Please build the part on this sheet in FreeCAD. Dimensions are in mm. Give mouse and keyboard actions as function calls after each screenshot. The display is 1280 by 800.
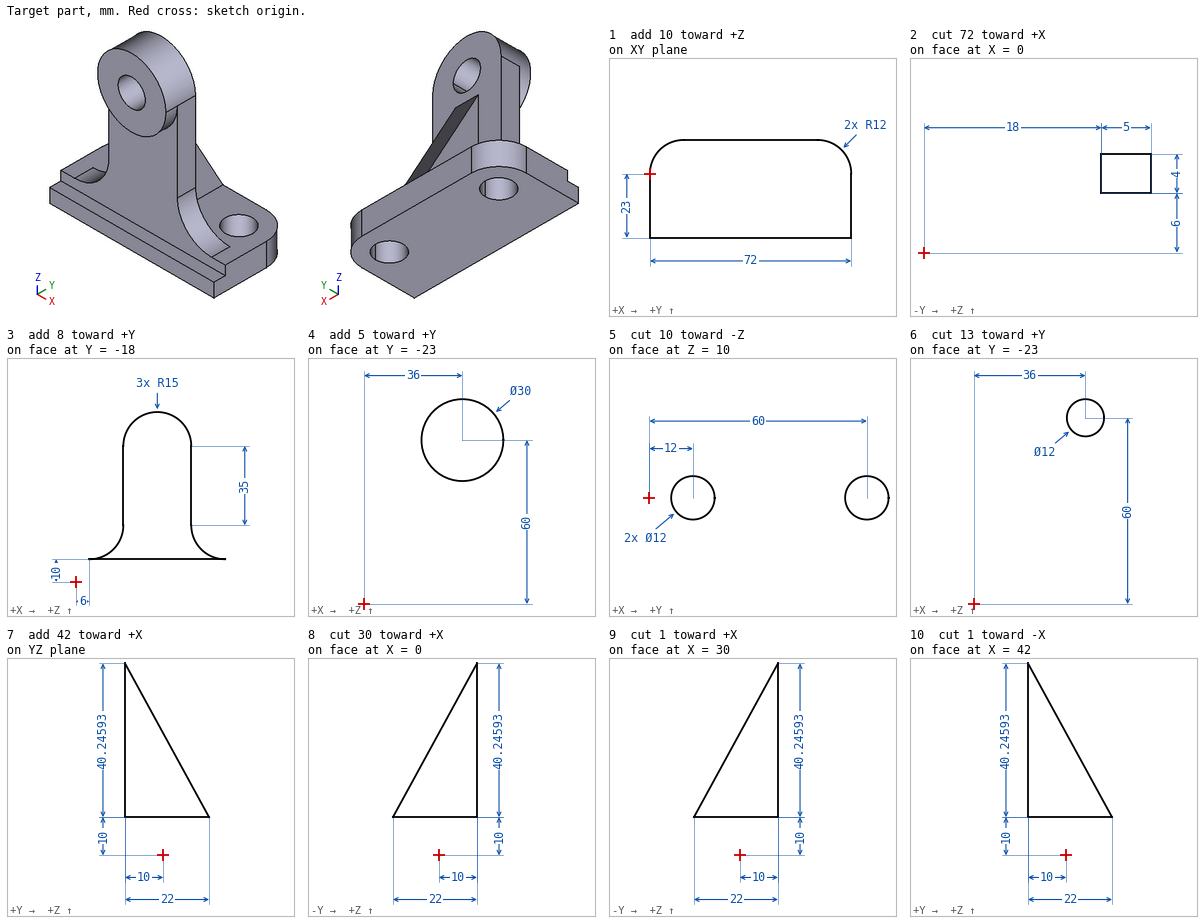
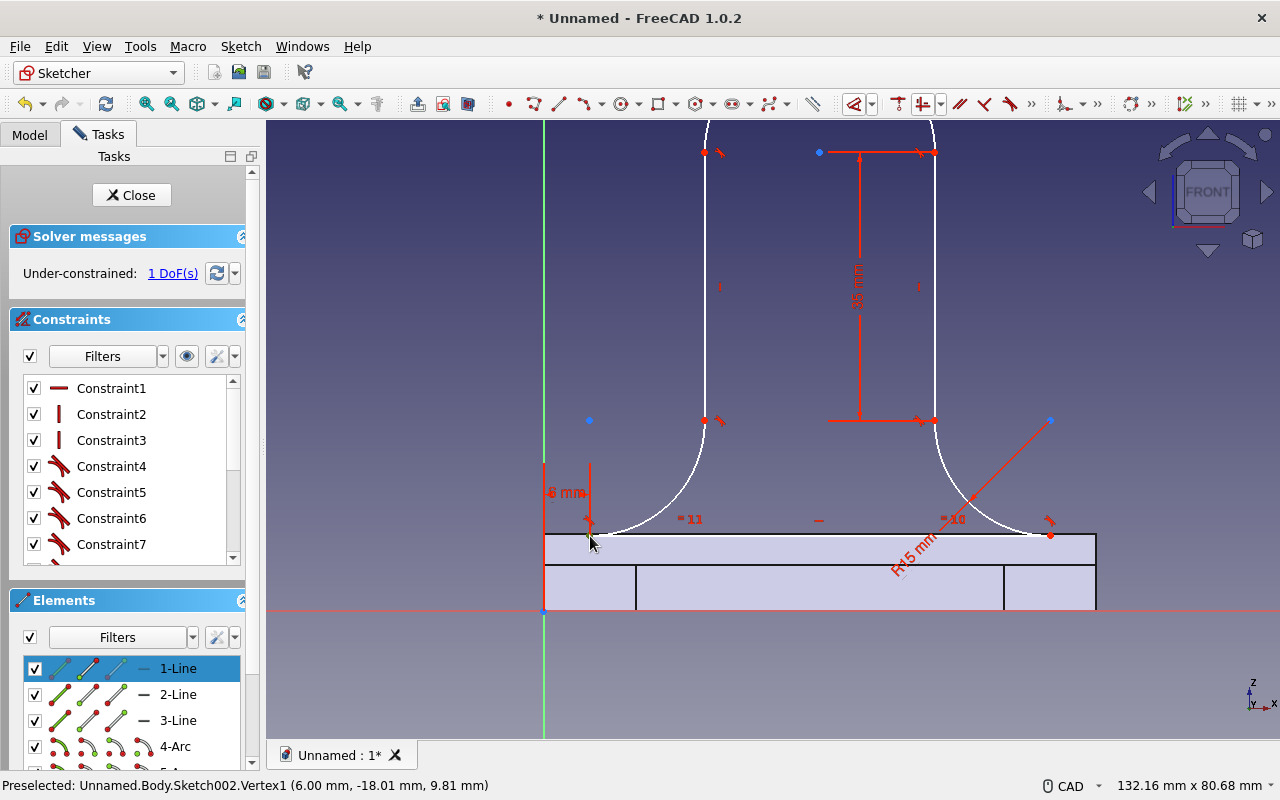
click(872, 104)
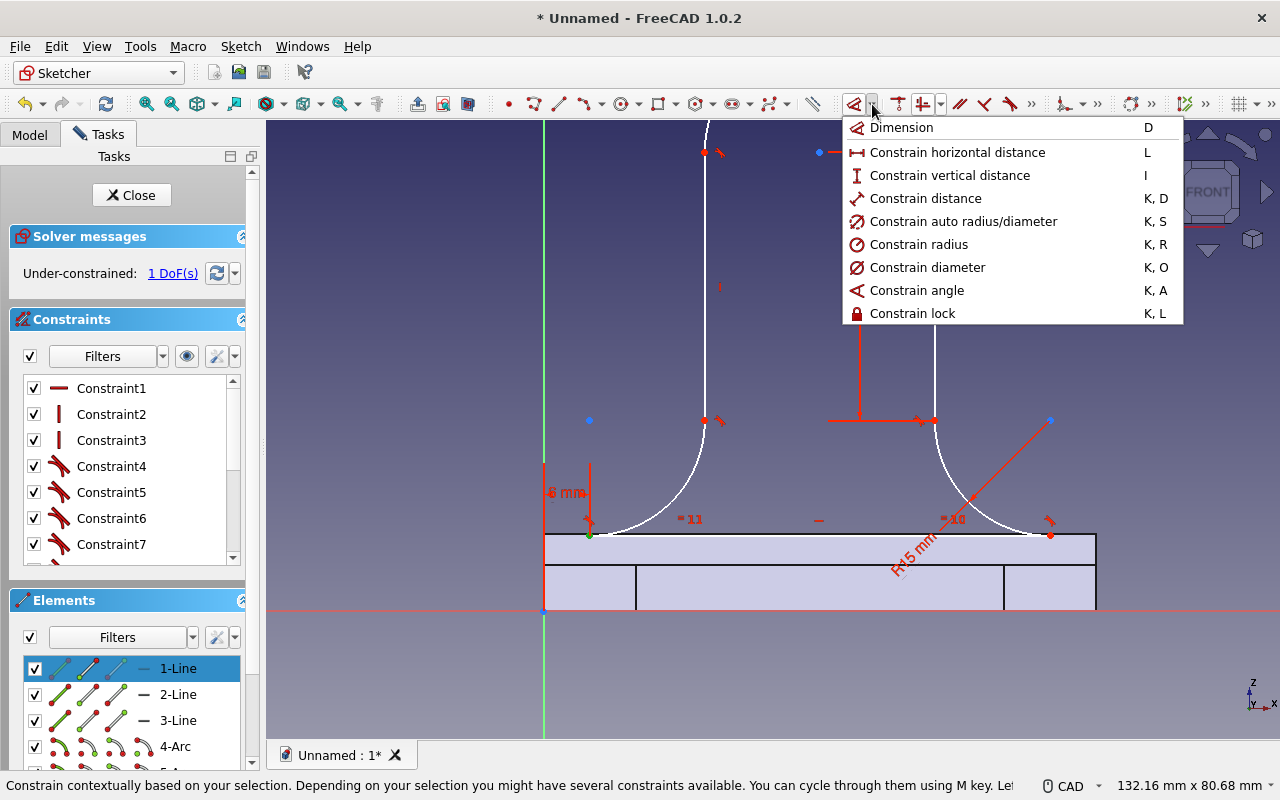
click(1013, 176)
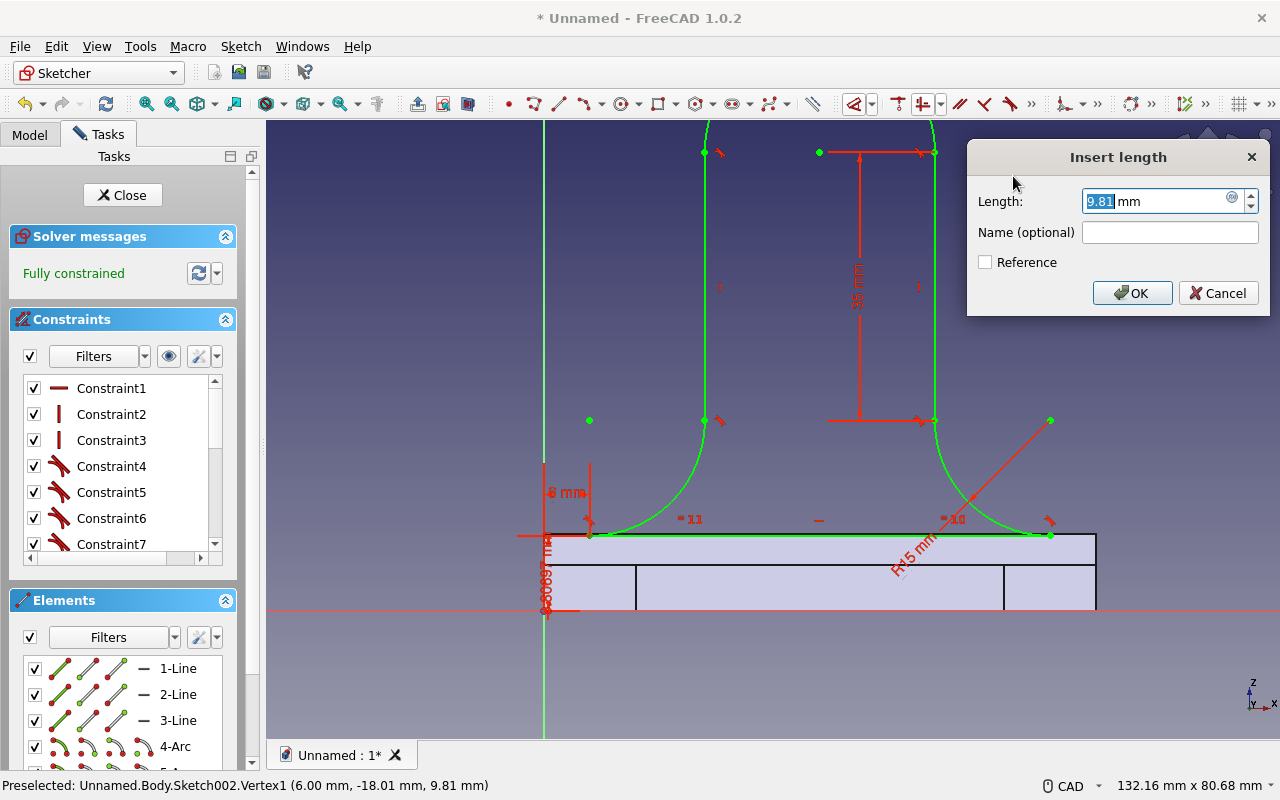
text(10)
key(Return)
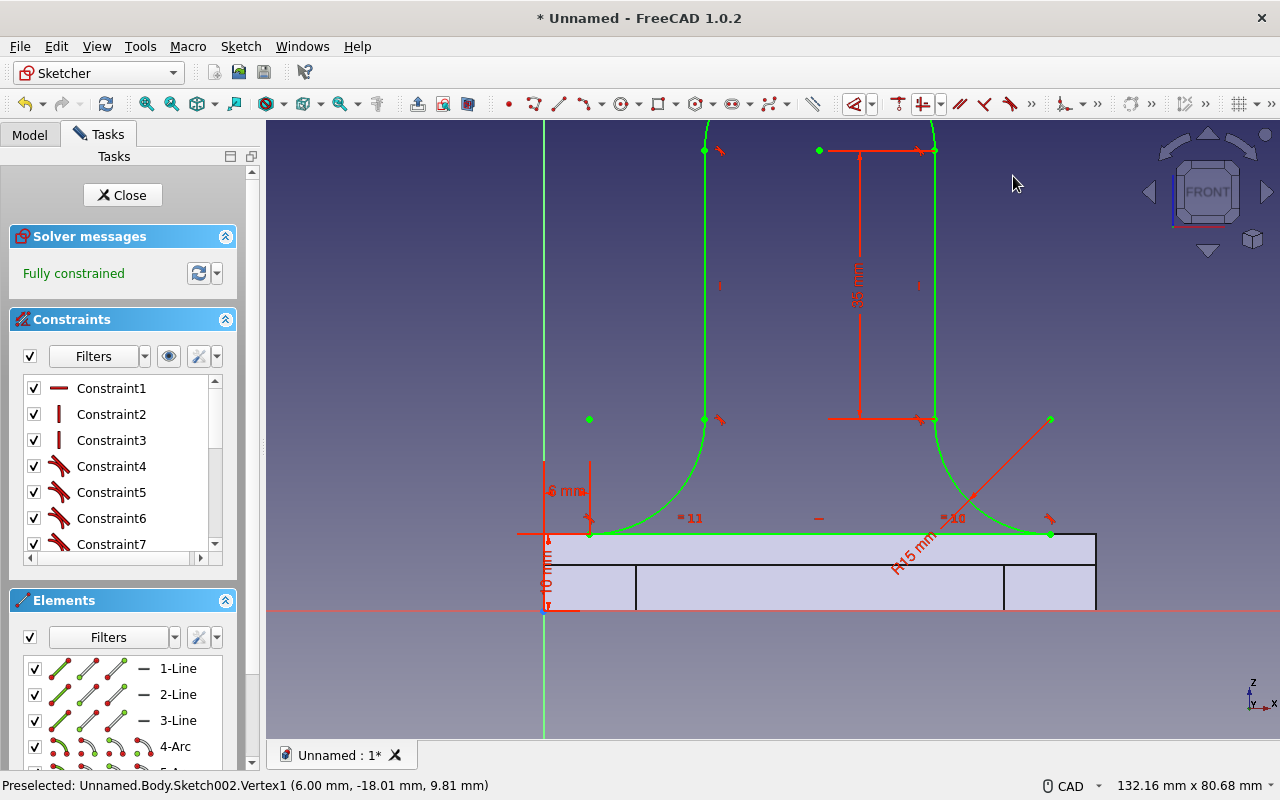
click(123, 195)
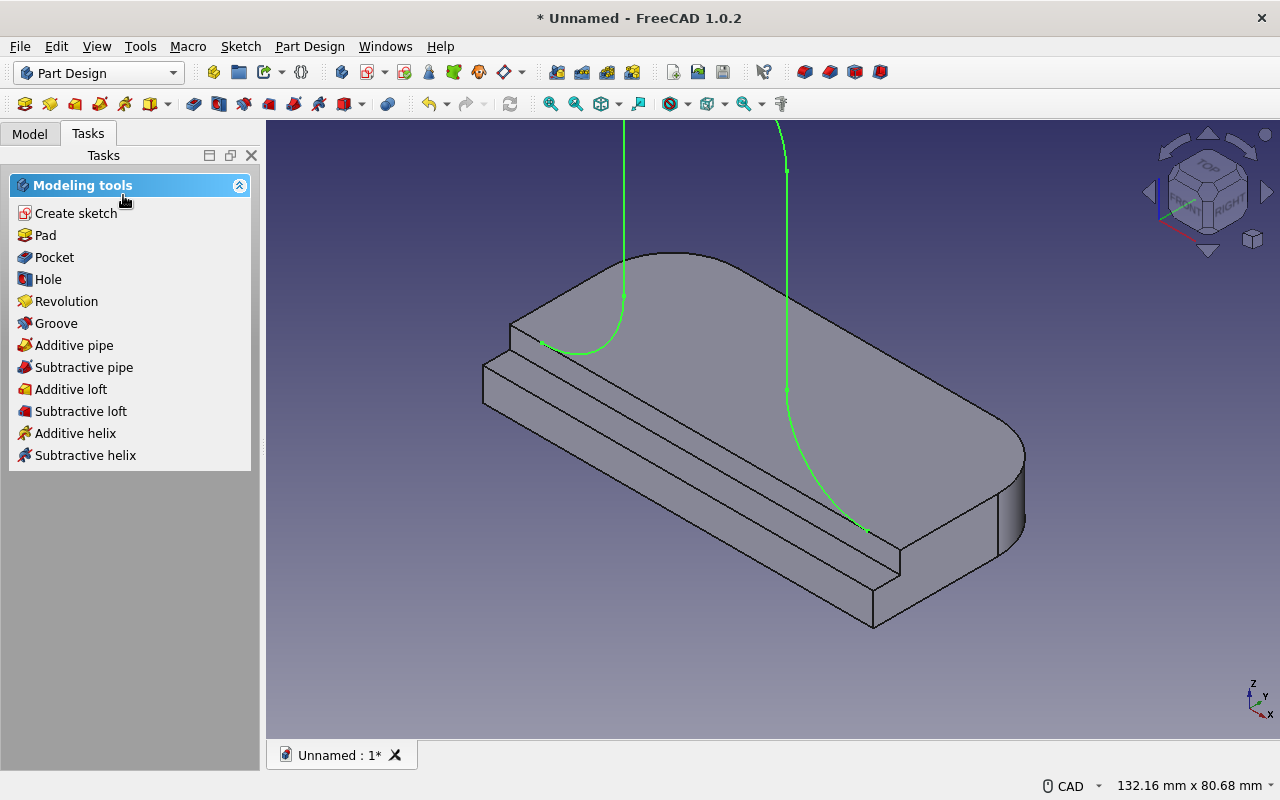
click(25, 104)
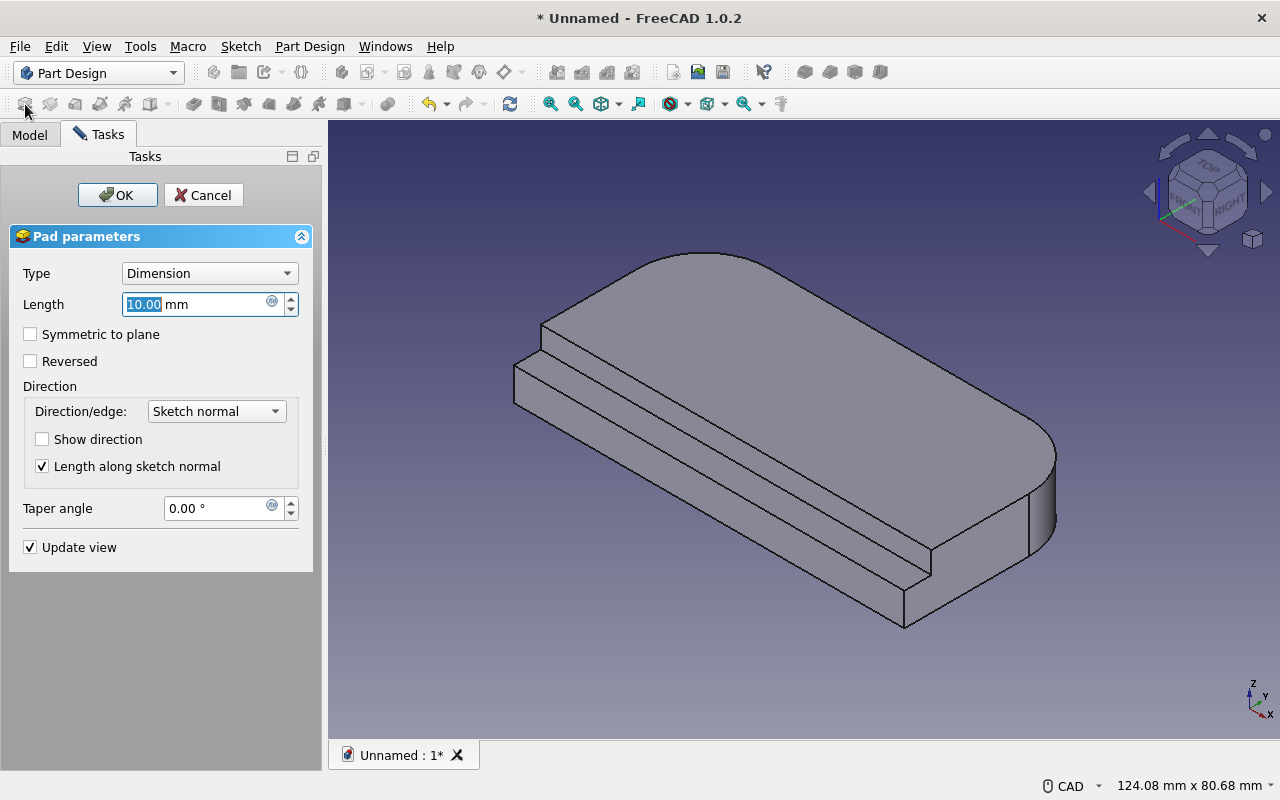
text(8)
key(Tab)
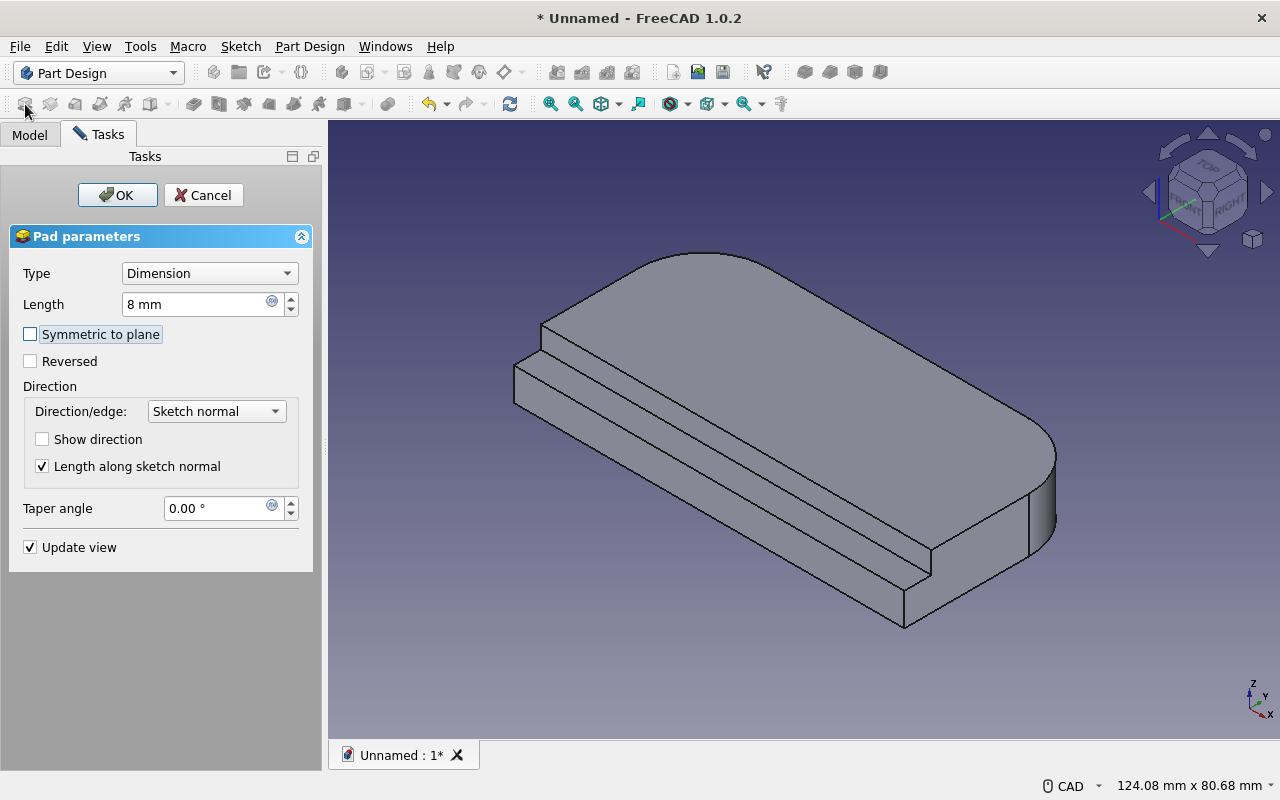
click(31, 361)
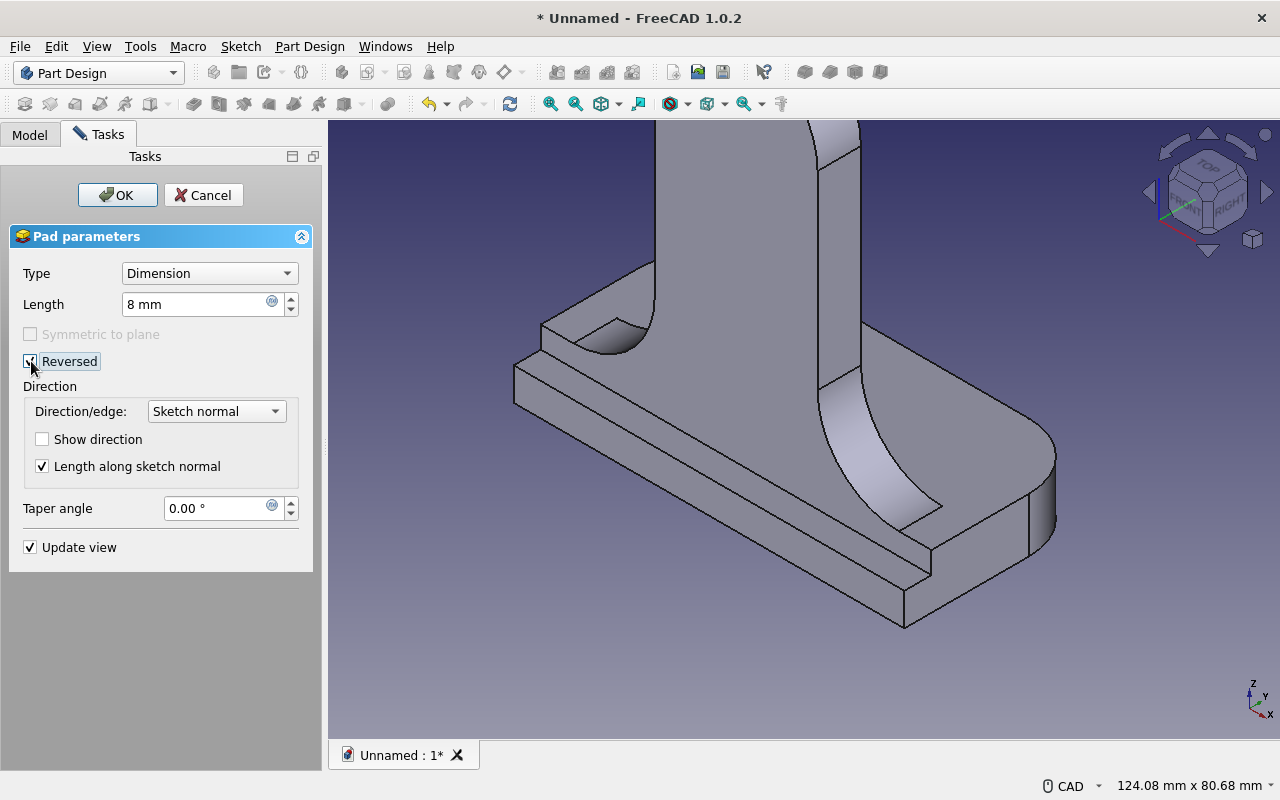
click(118, 195)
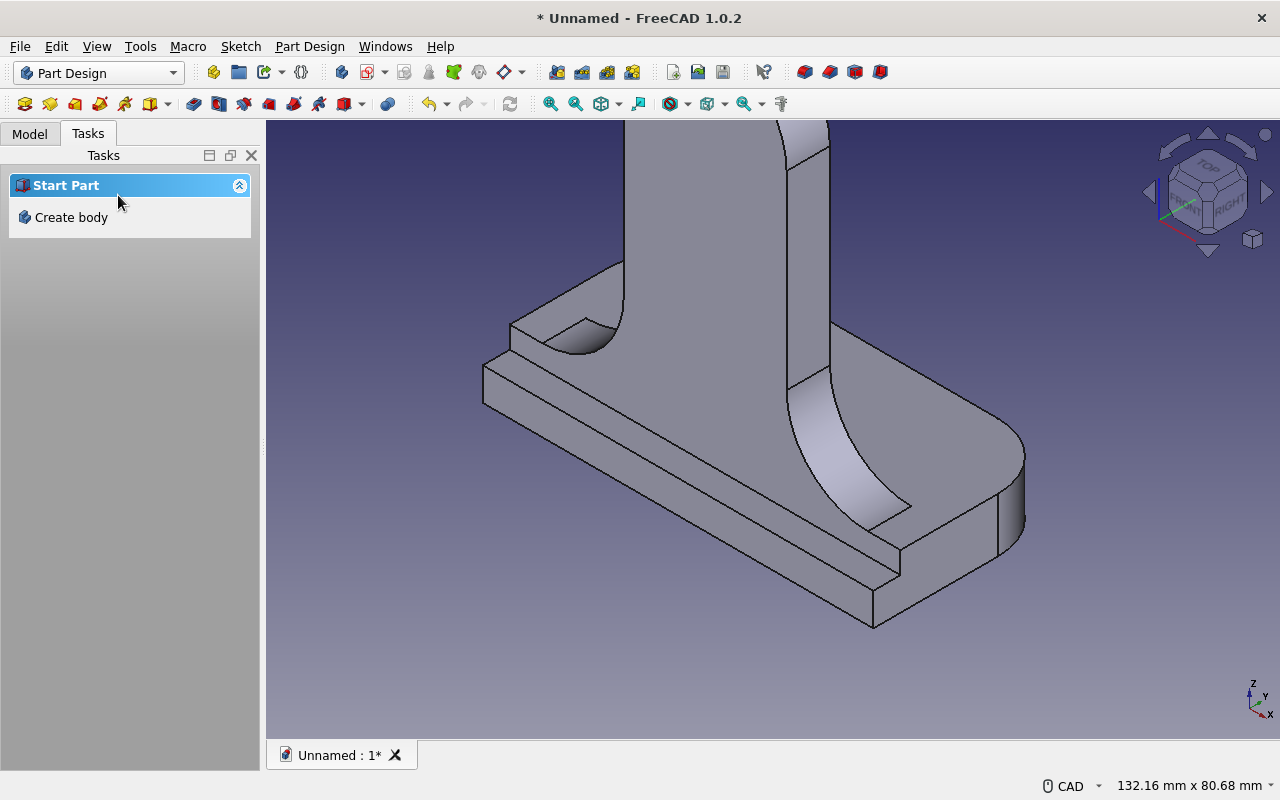
click(551, 104)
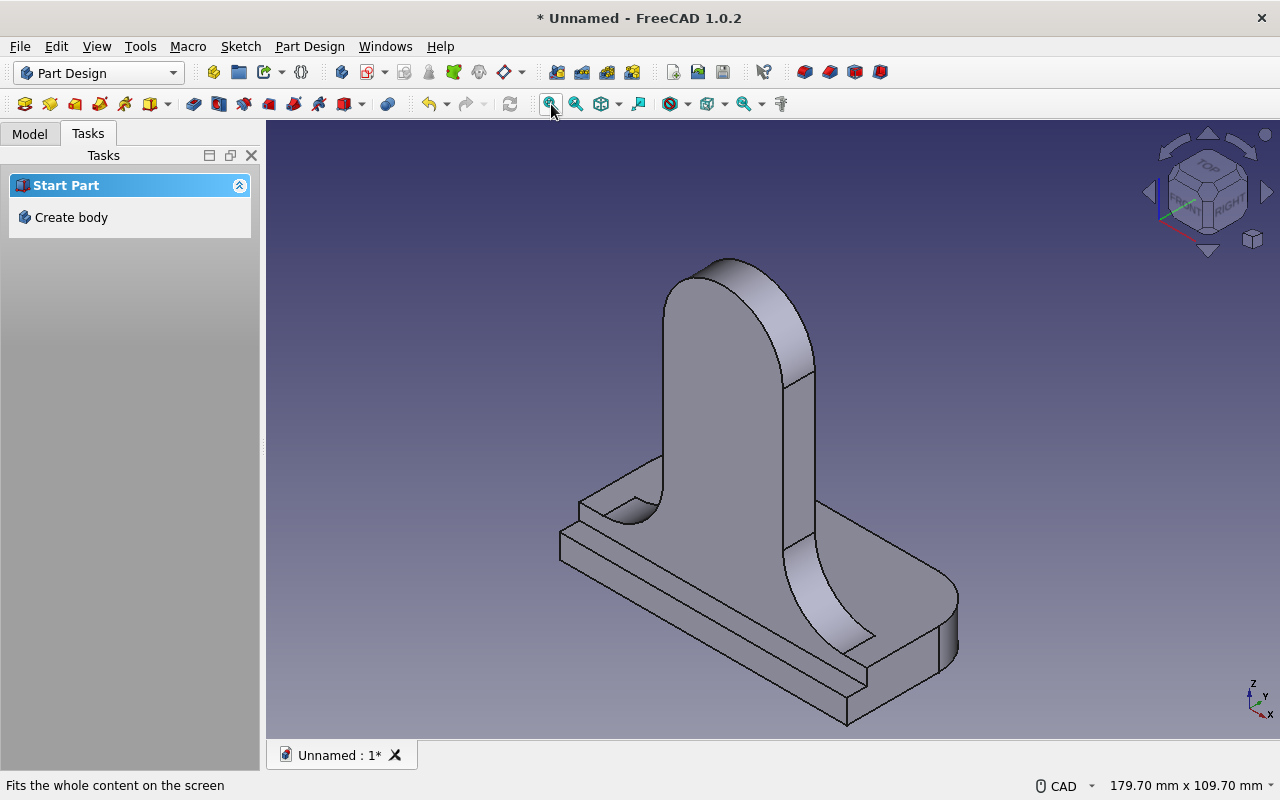
click(826, 699)